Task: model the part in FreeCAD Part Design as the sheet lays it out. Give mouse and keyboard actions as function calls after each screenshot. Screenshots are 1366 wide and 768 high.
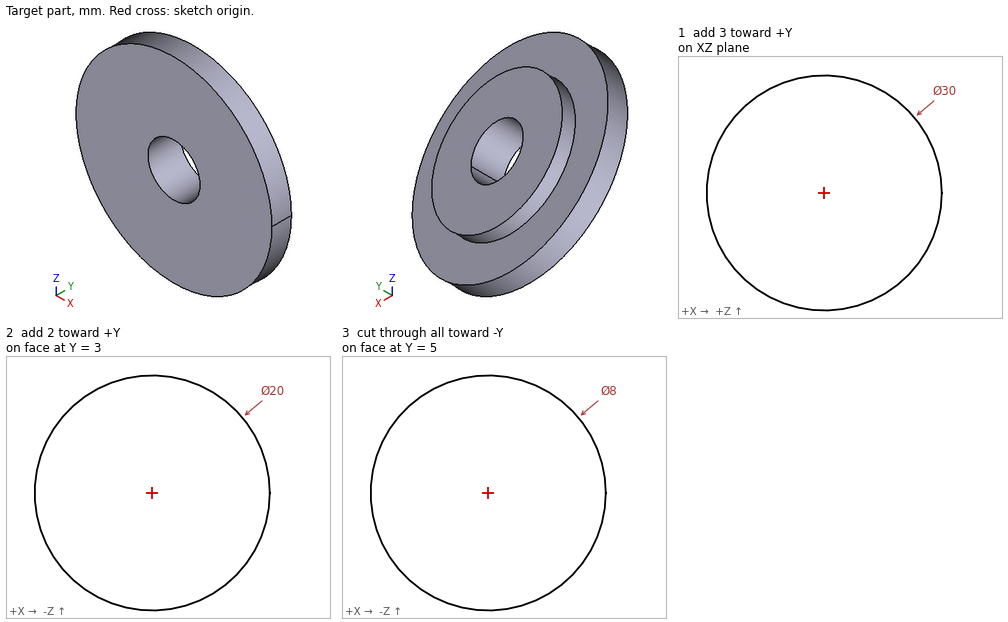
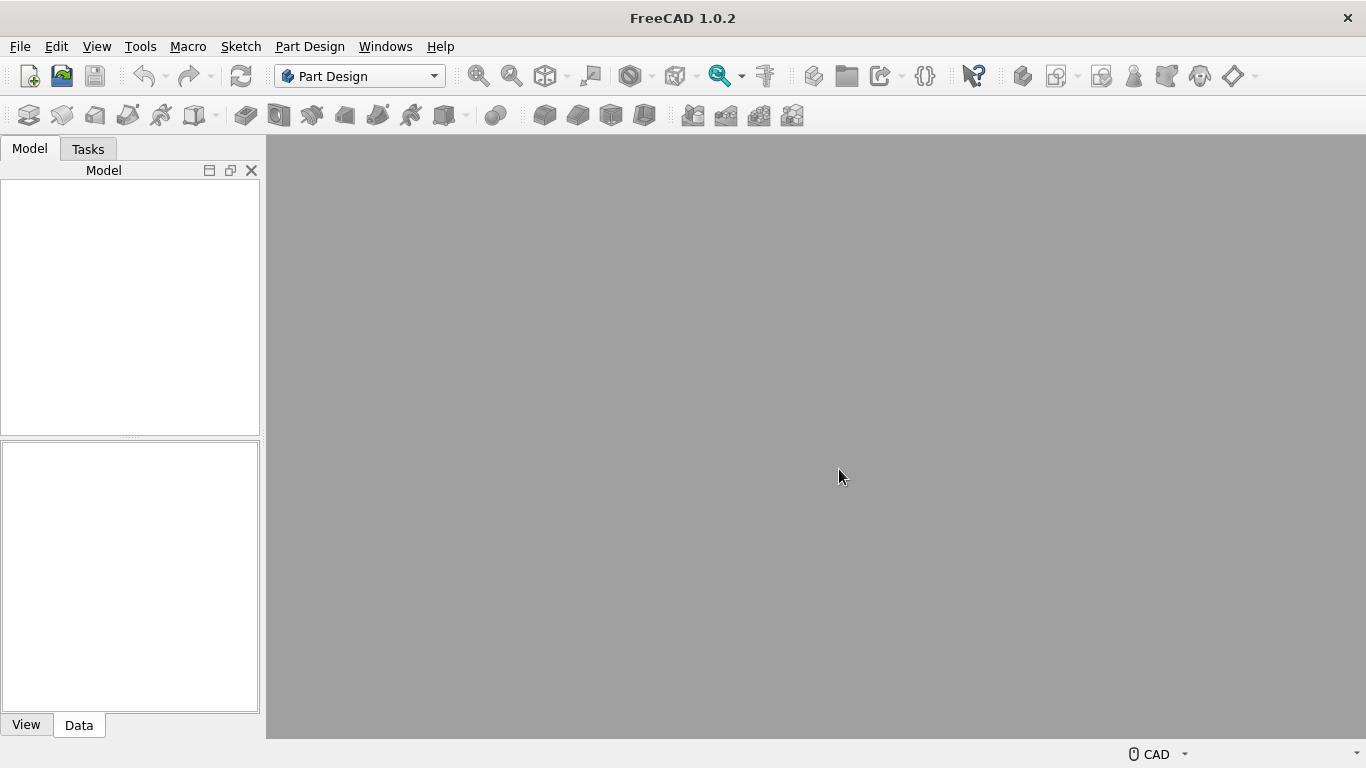
click(29, 76)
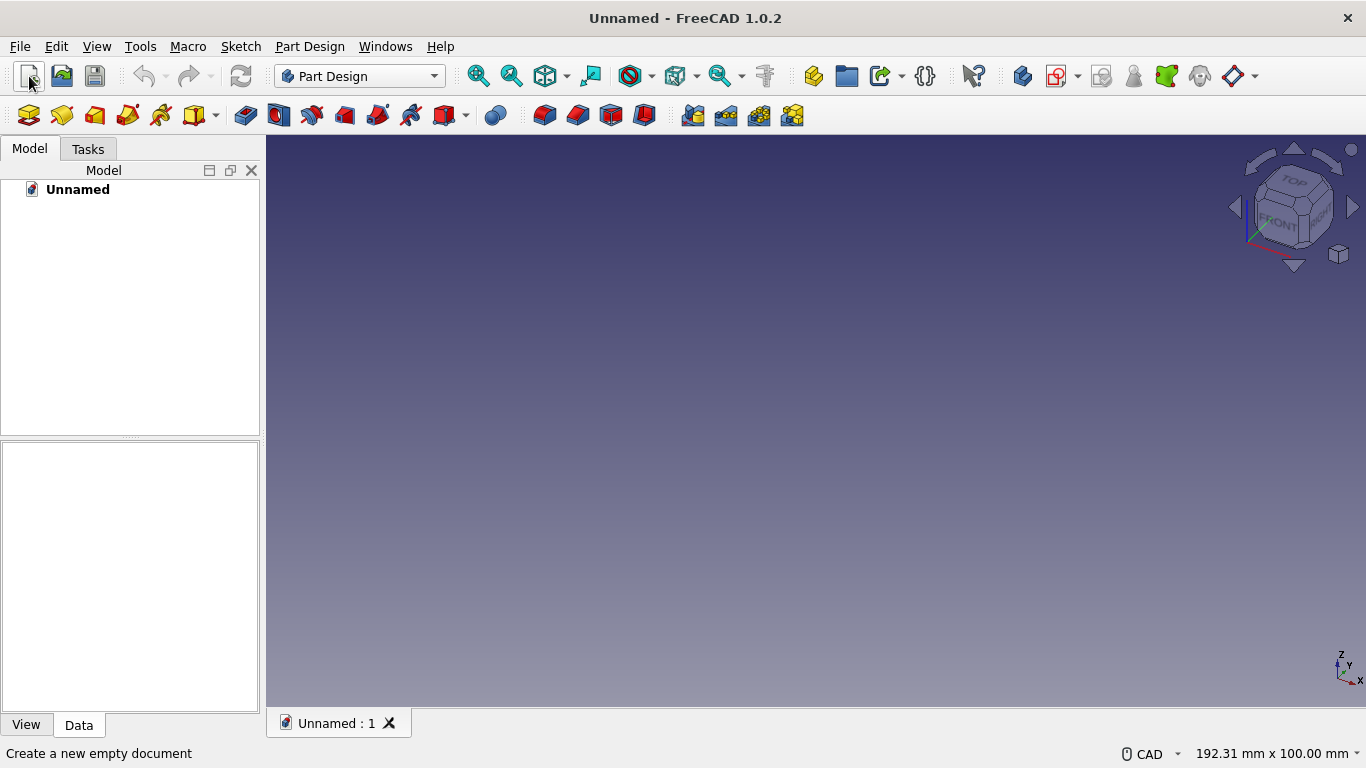
click(1056, 76)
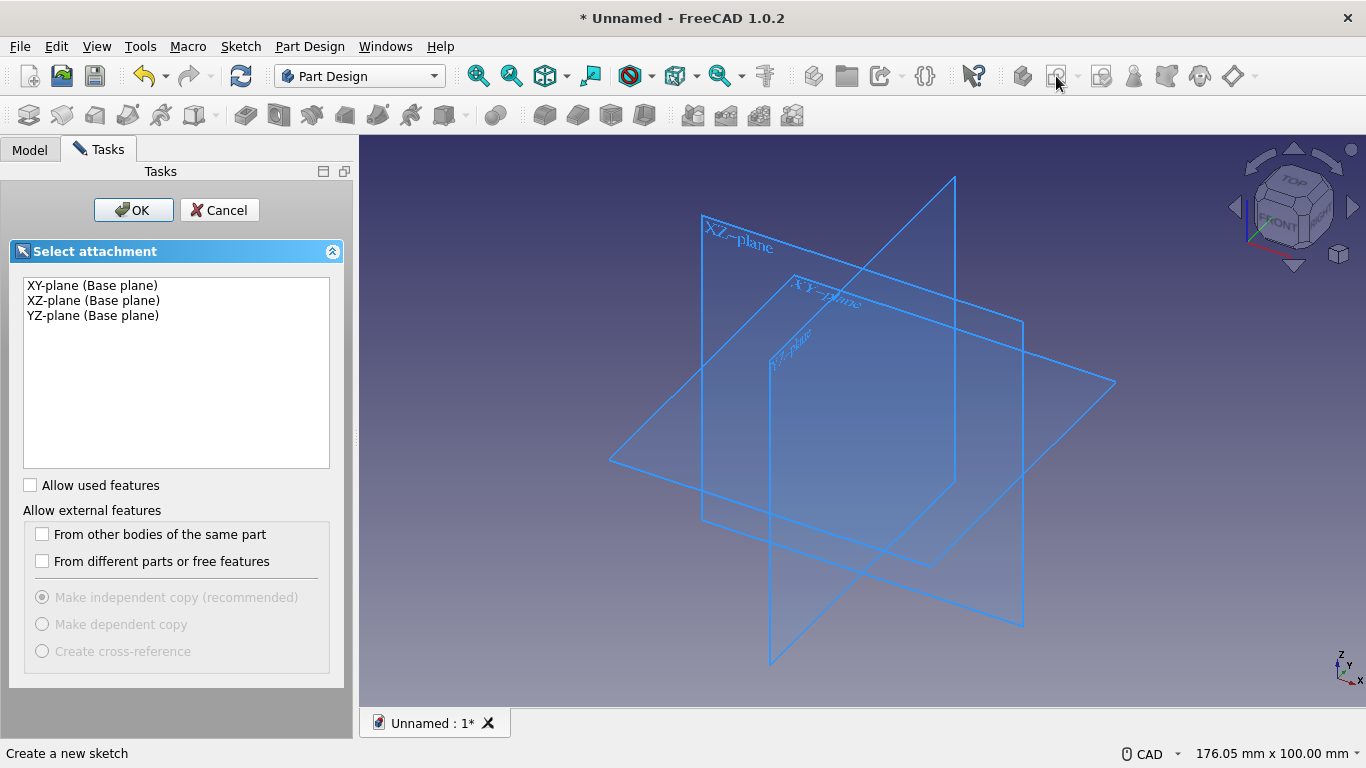
click(84, 300)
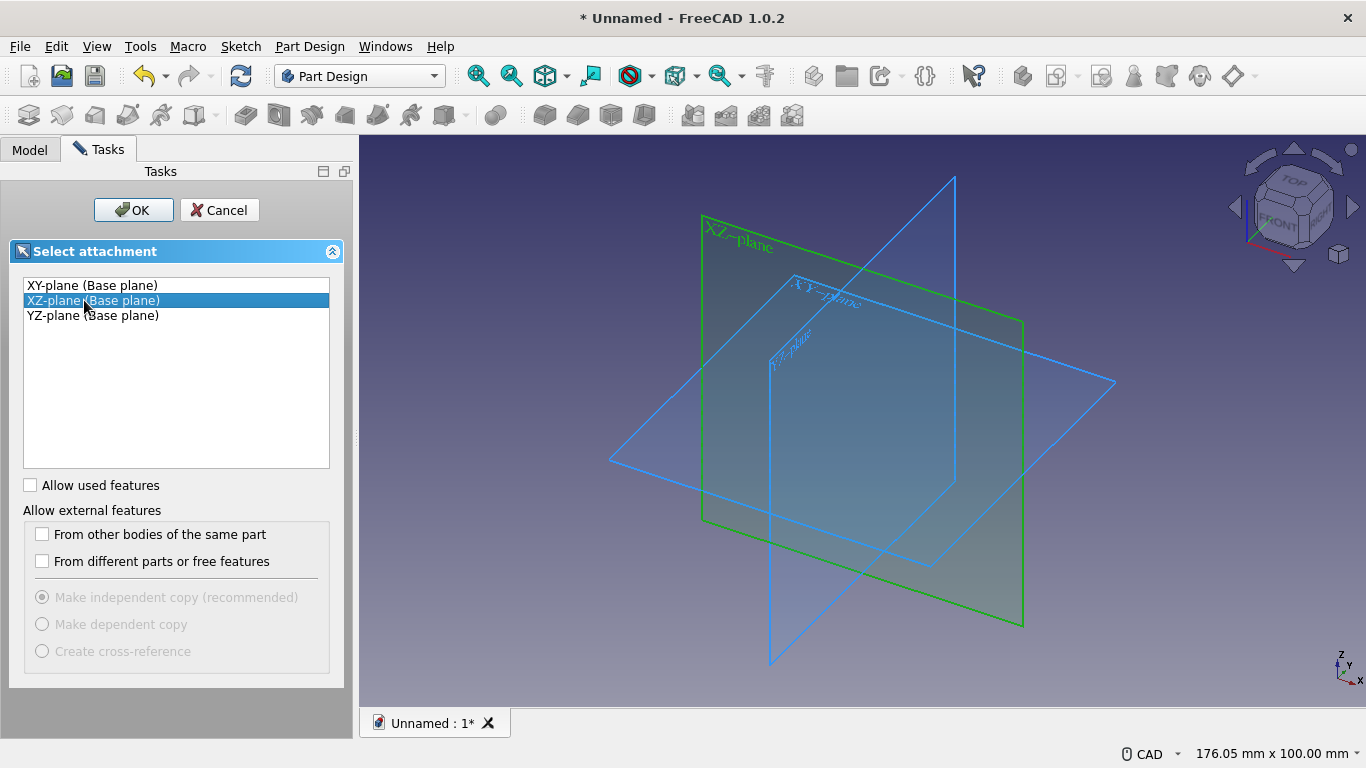
click(134, 210)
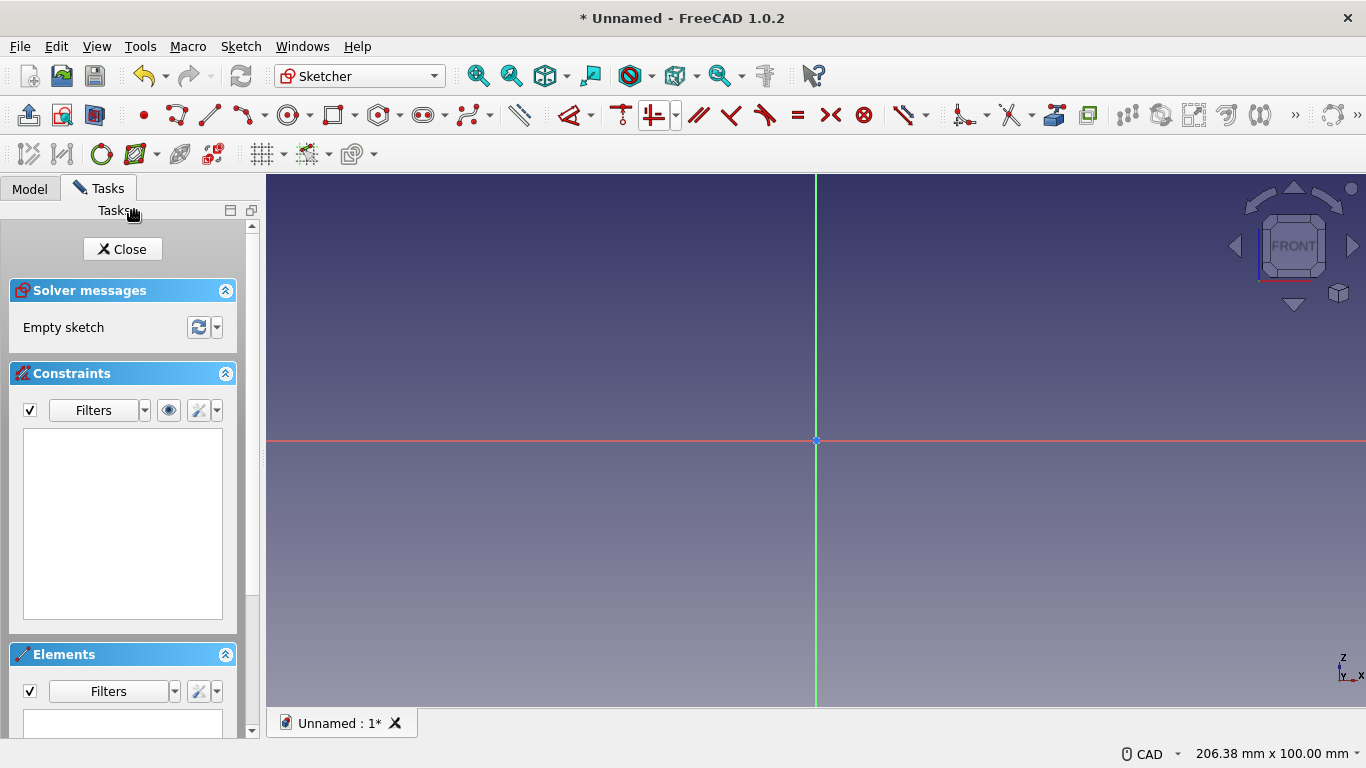
scroll(872, 440, up, 4)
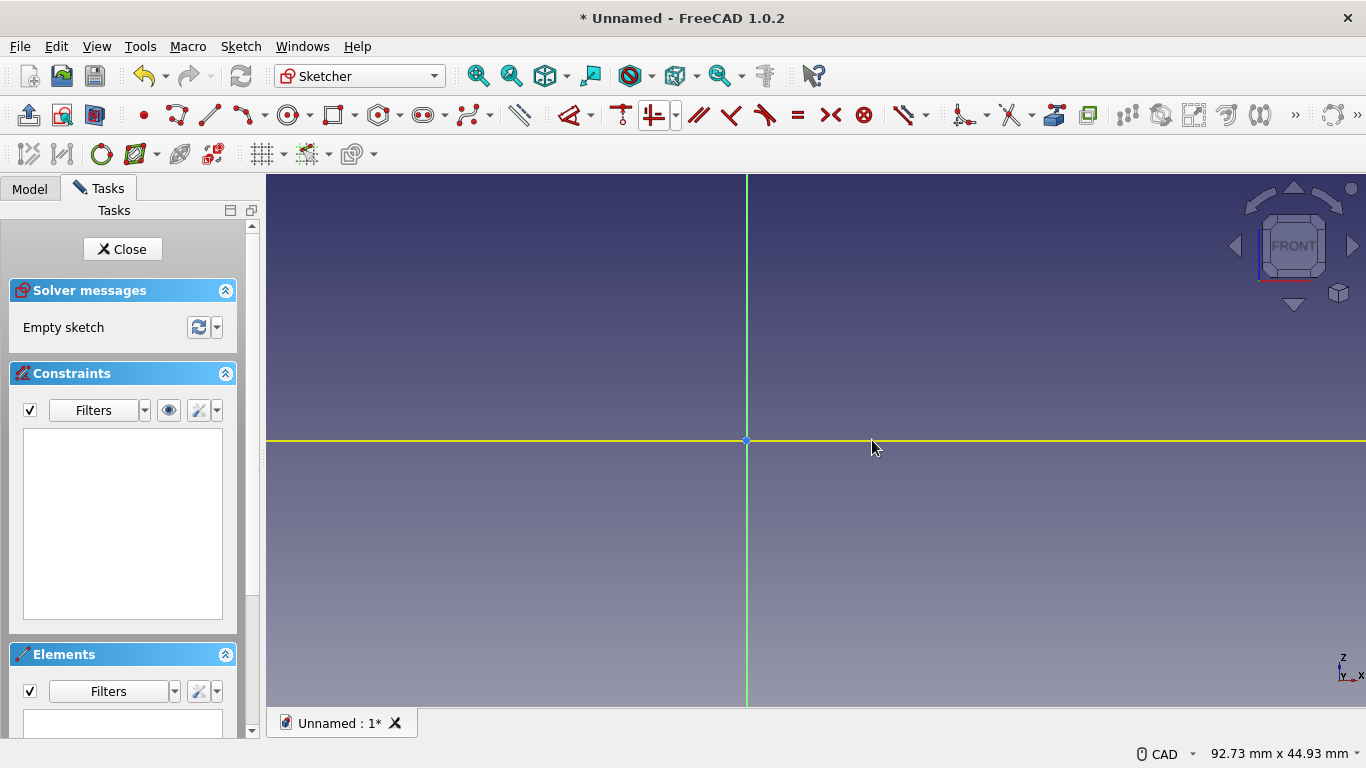
click(288, 116)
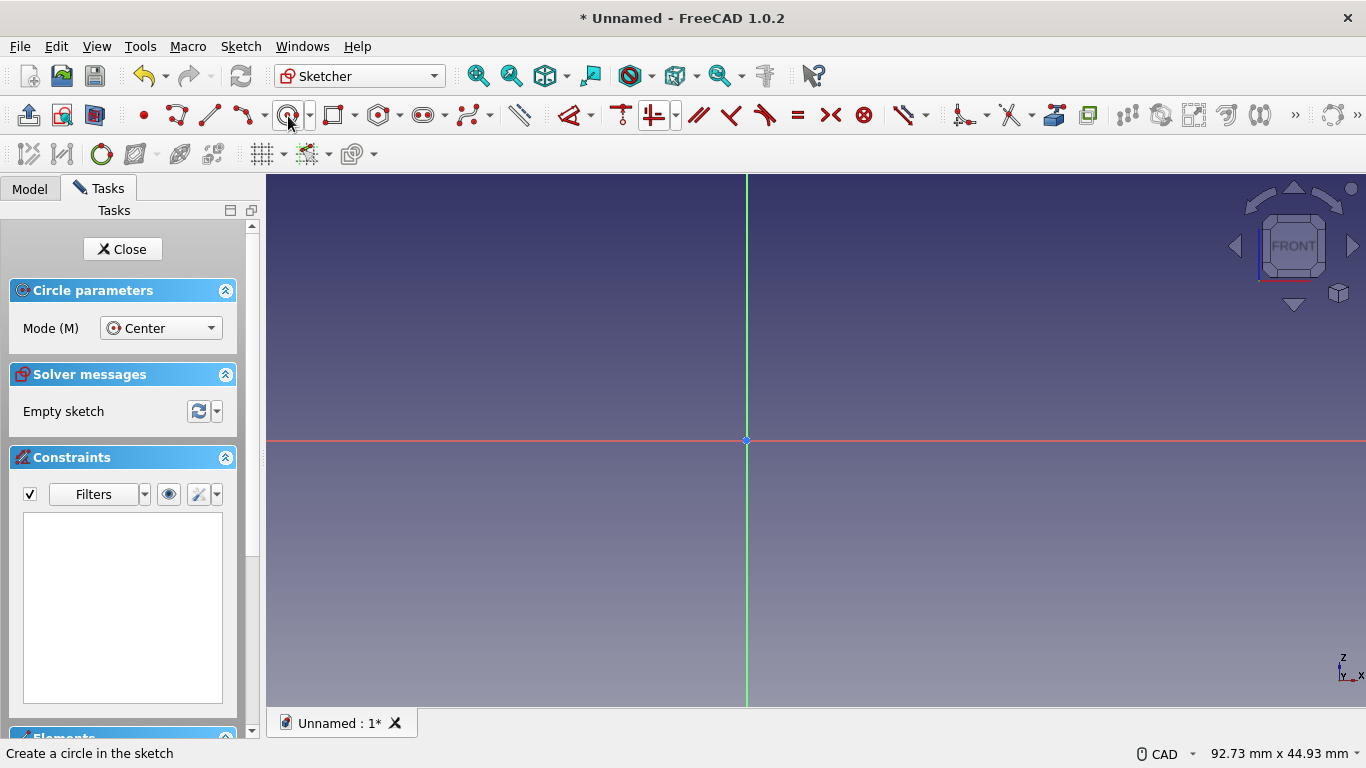
click(747, 440)
click(873, 315)
key(Escape)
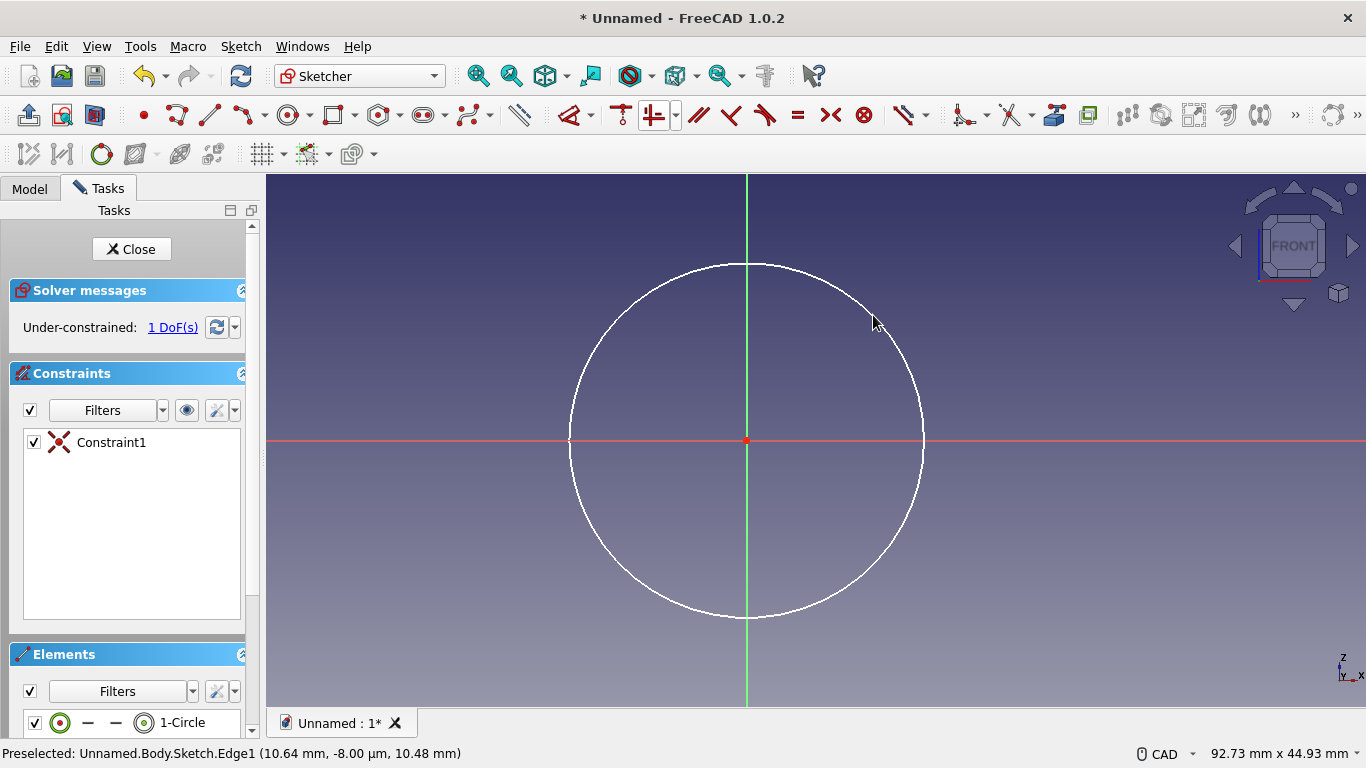
click(568, 116)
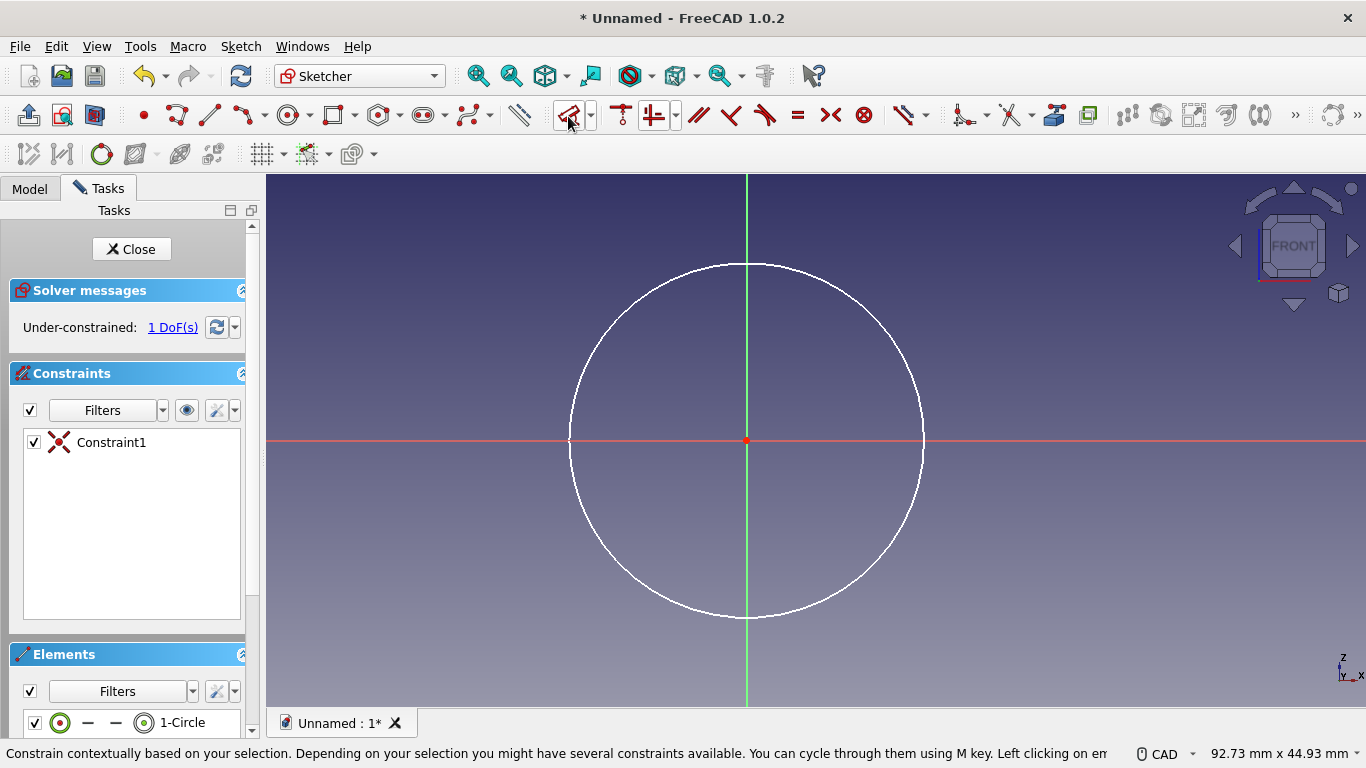
click(872, 315)
click(895, 292)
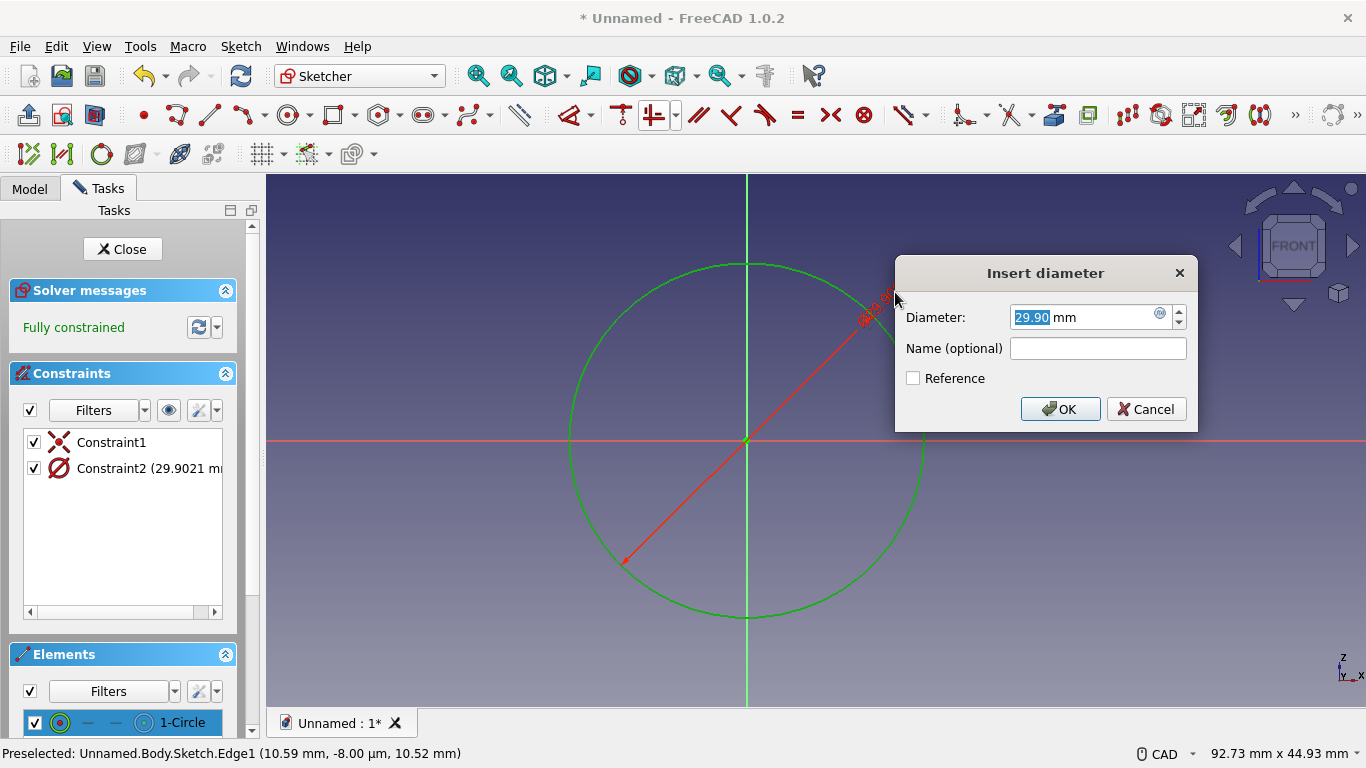
text(30)
key(Return)
key(Escape)